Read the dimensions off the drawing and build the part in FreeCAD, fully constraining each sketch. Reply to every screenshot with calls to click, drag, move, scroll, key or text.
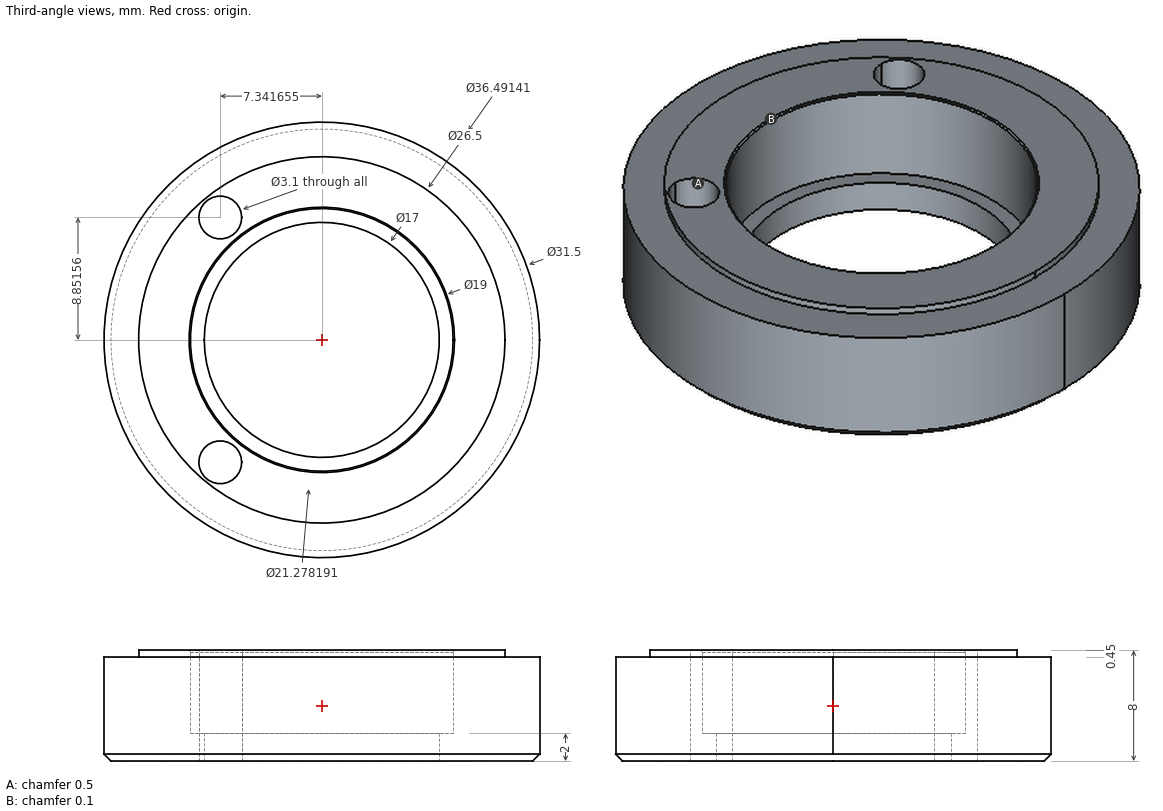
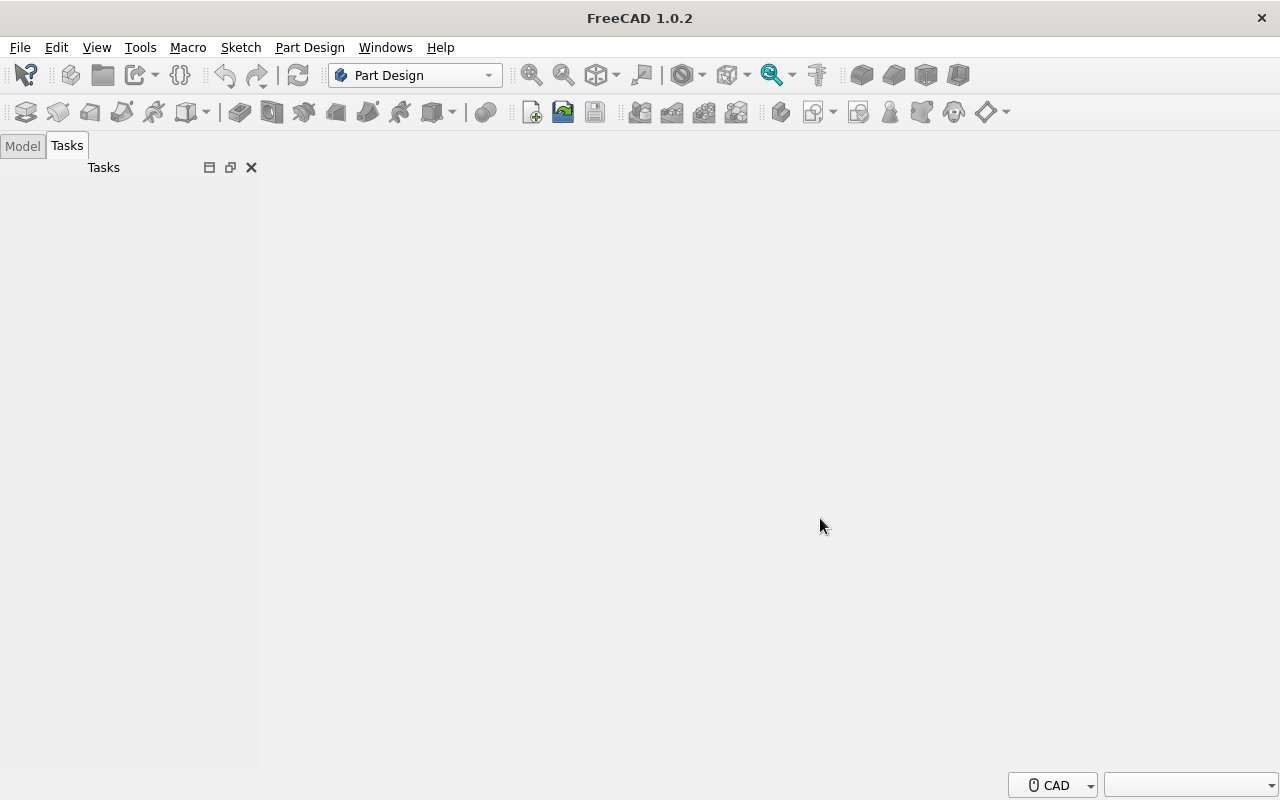
click(532, 112)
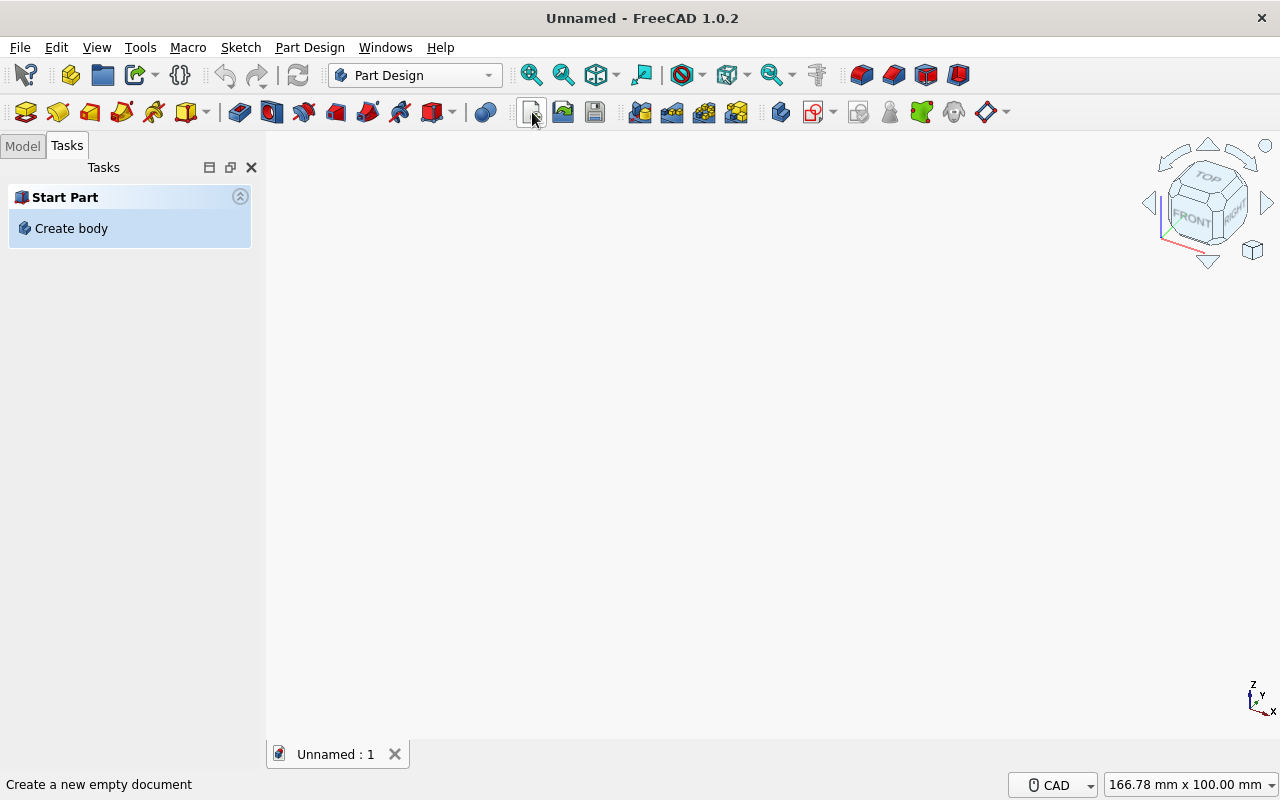
click(814, 112)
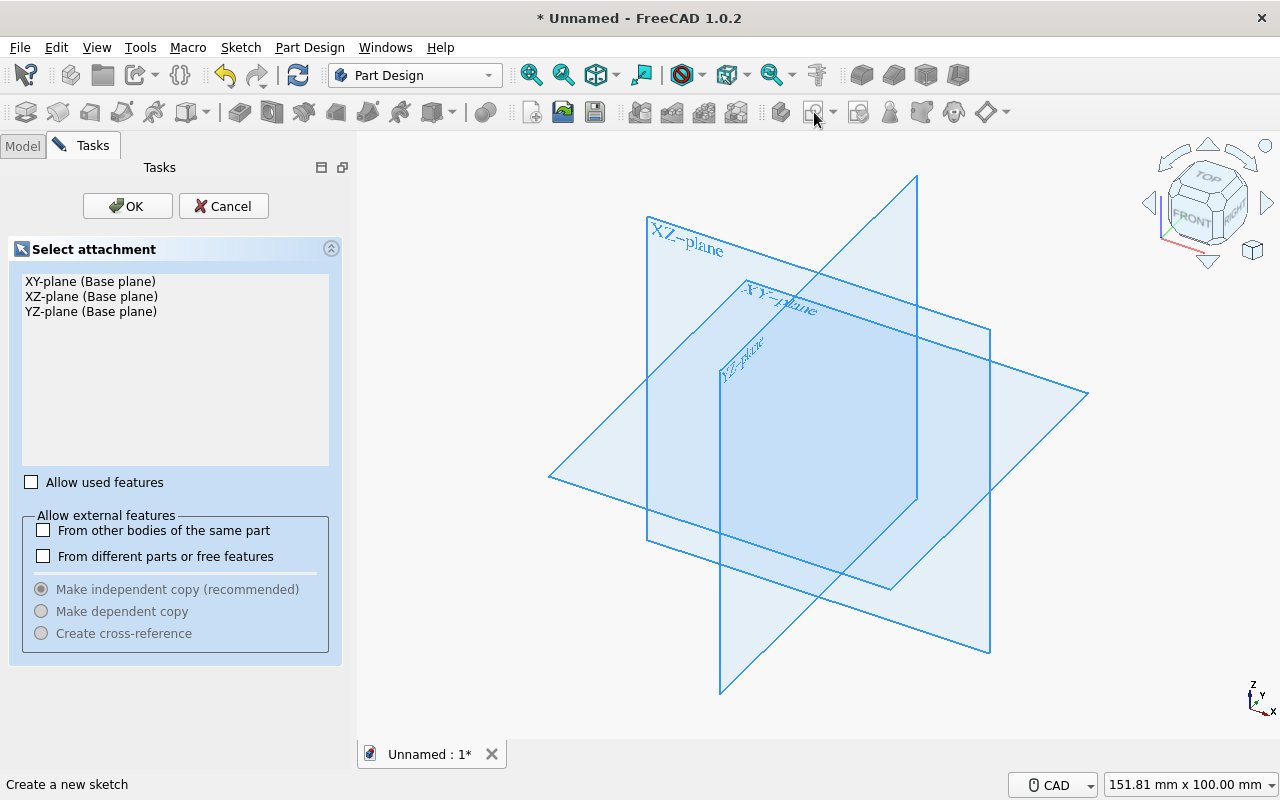
click(82, 282)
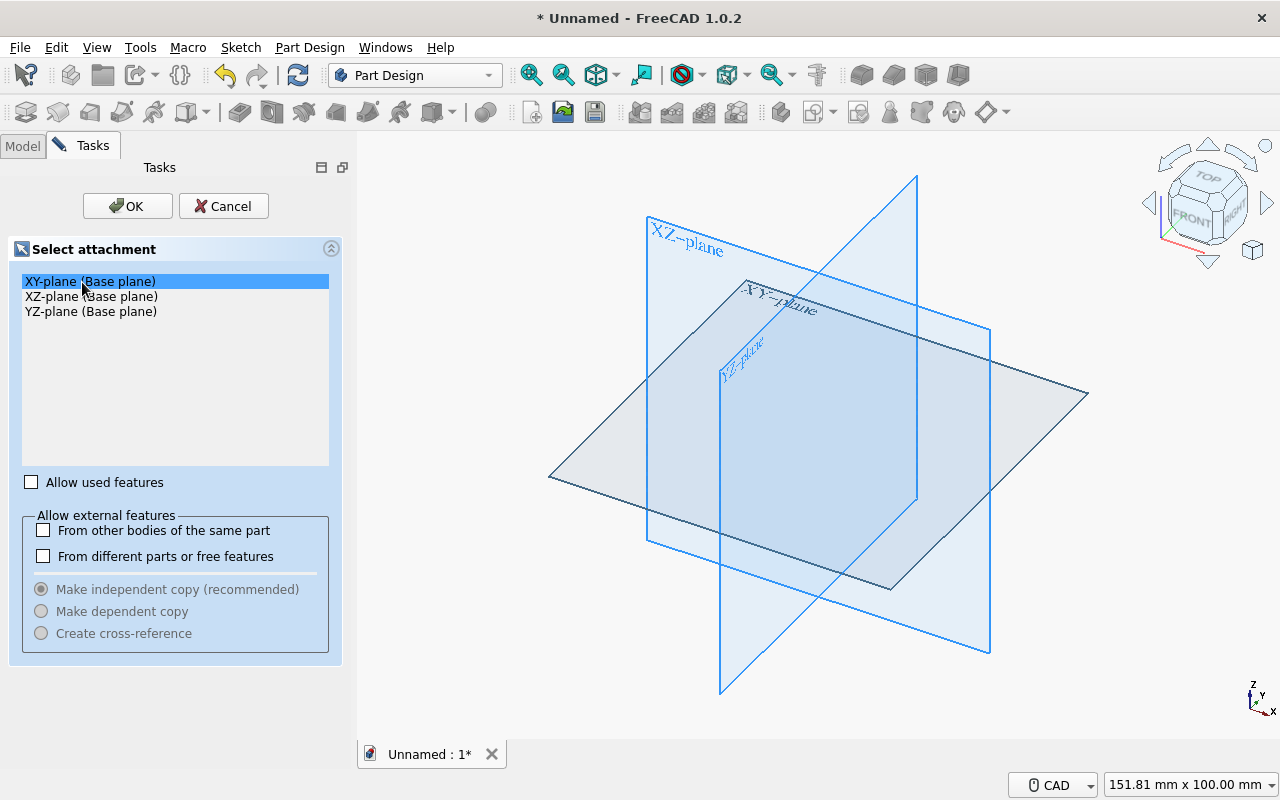
click(128, 206)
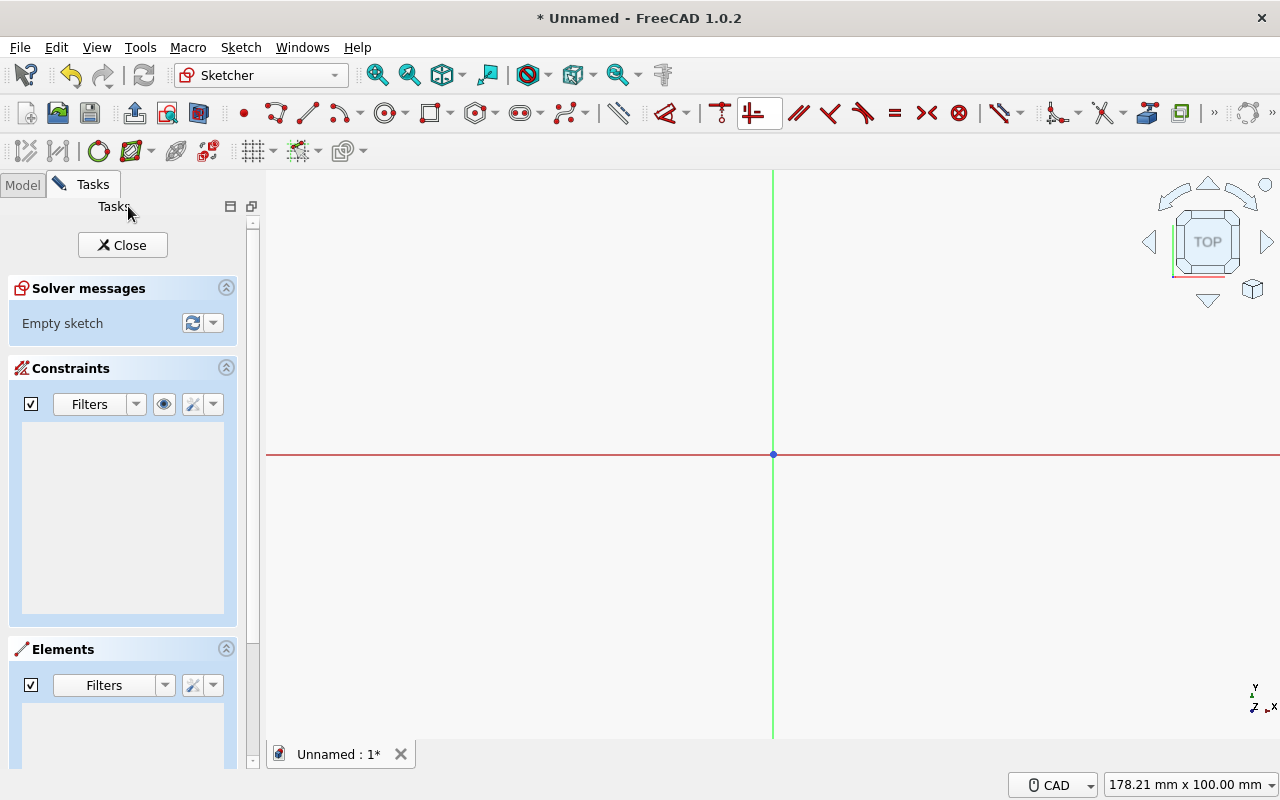
scroll(829, 455, up, 4)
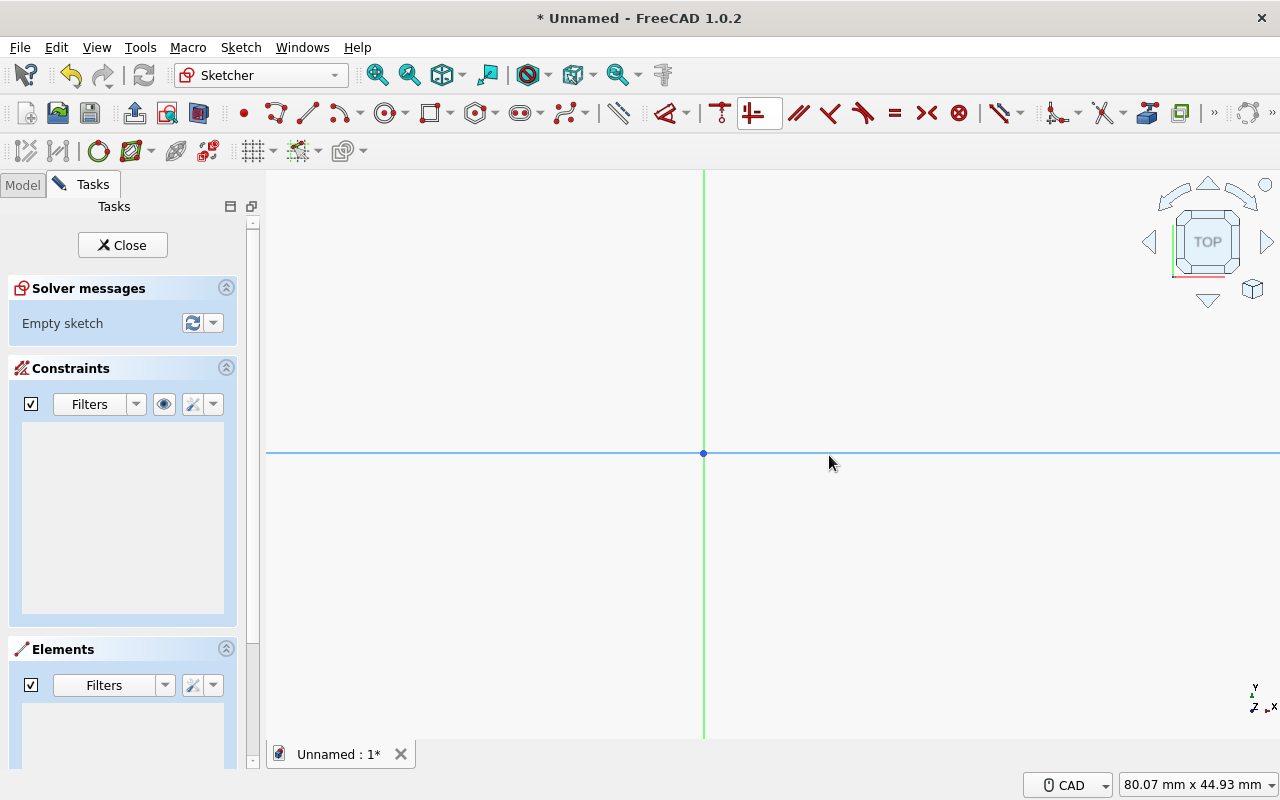
key(g)
key(c)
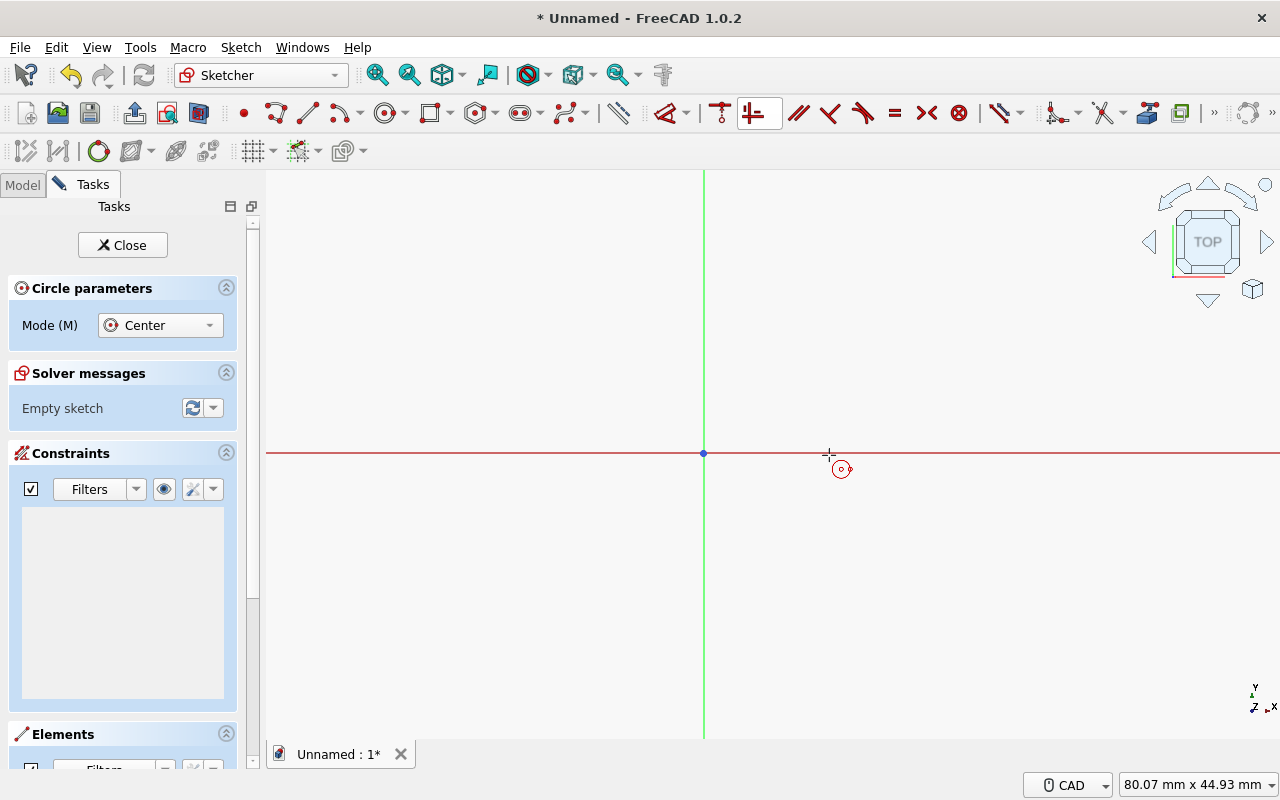
click(704, 453)
move(845, 312)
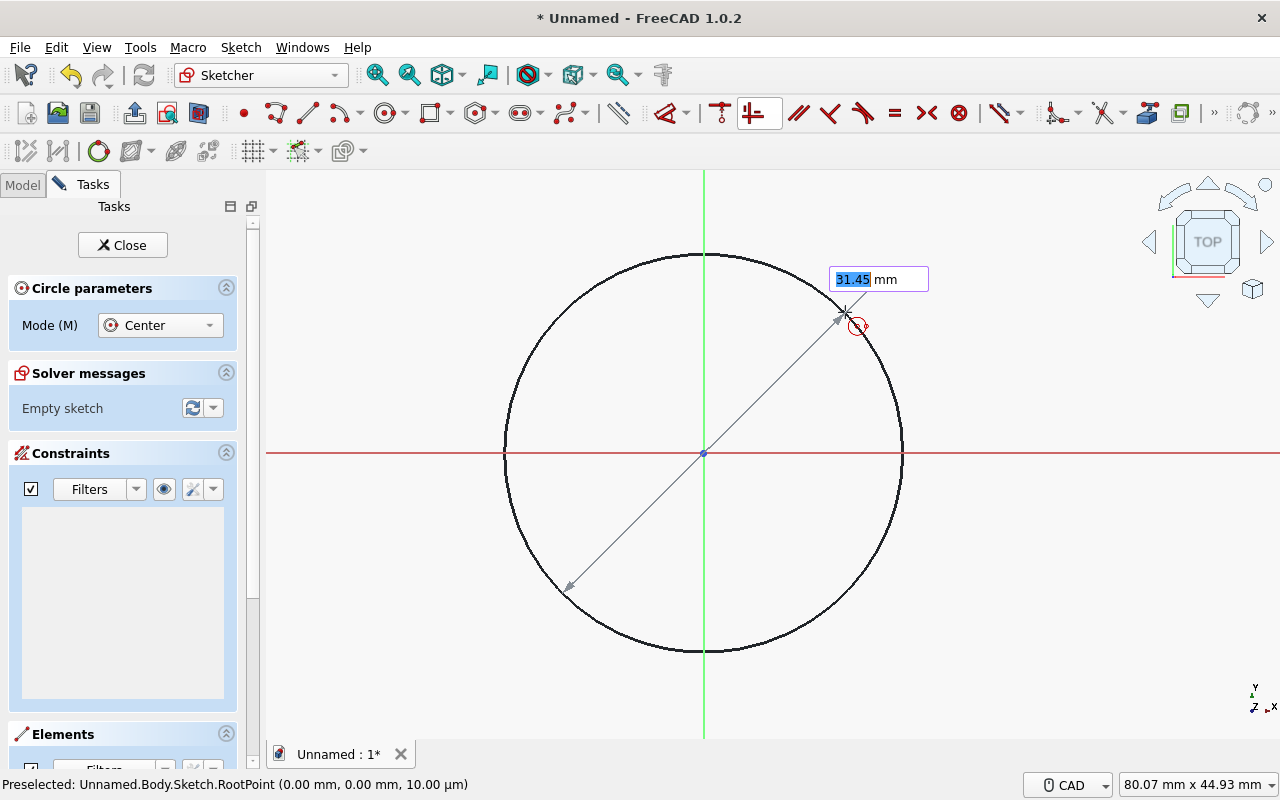
text(31.5)
key(Return)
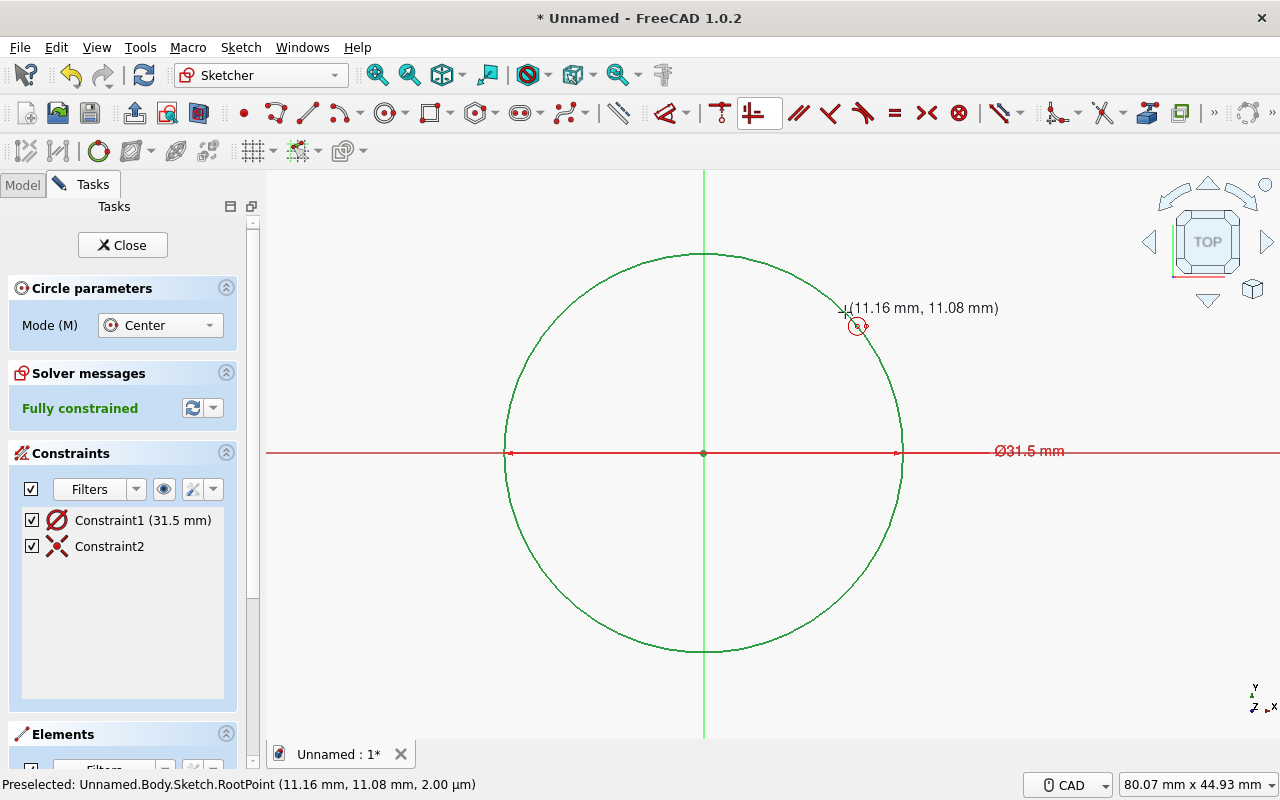
click(704, 453)
move(789, 368)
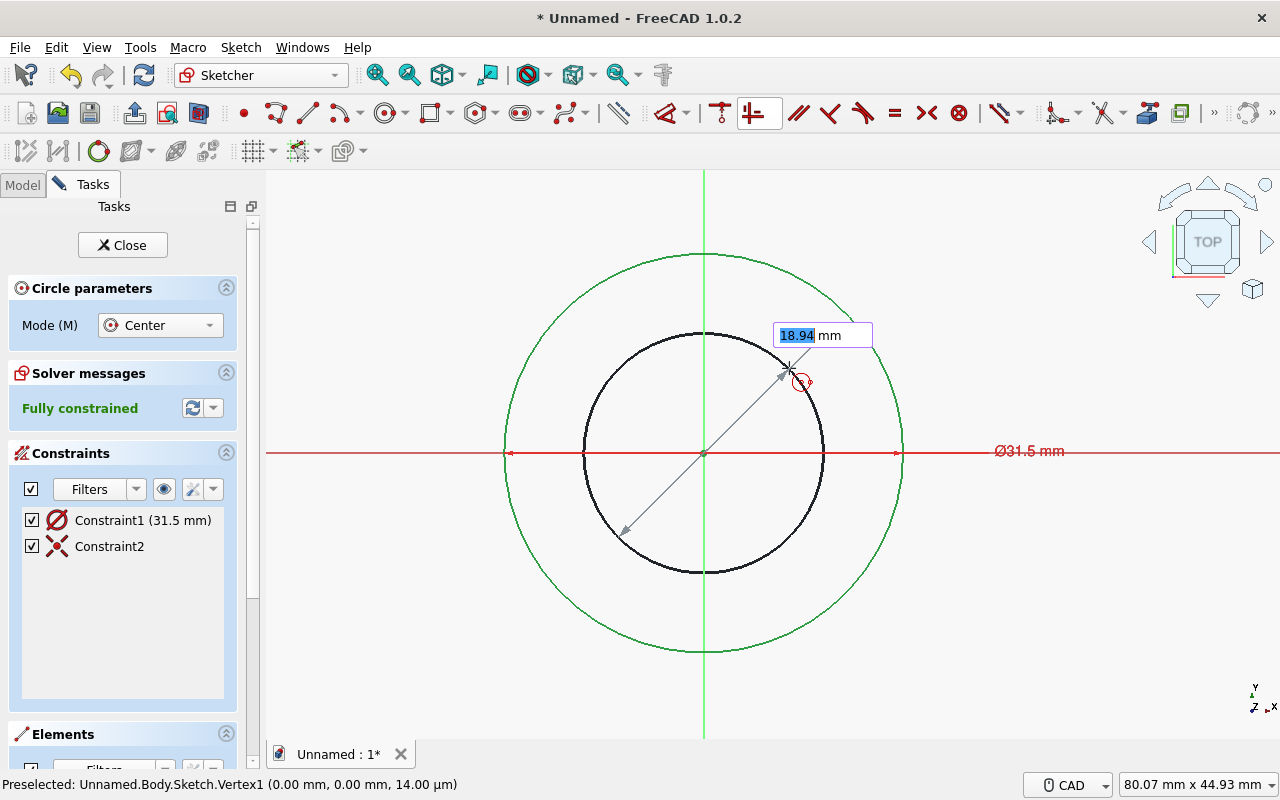
text(19)
key(Return)
key(Escape)